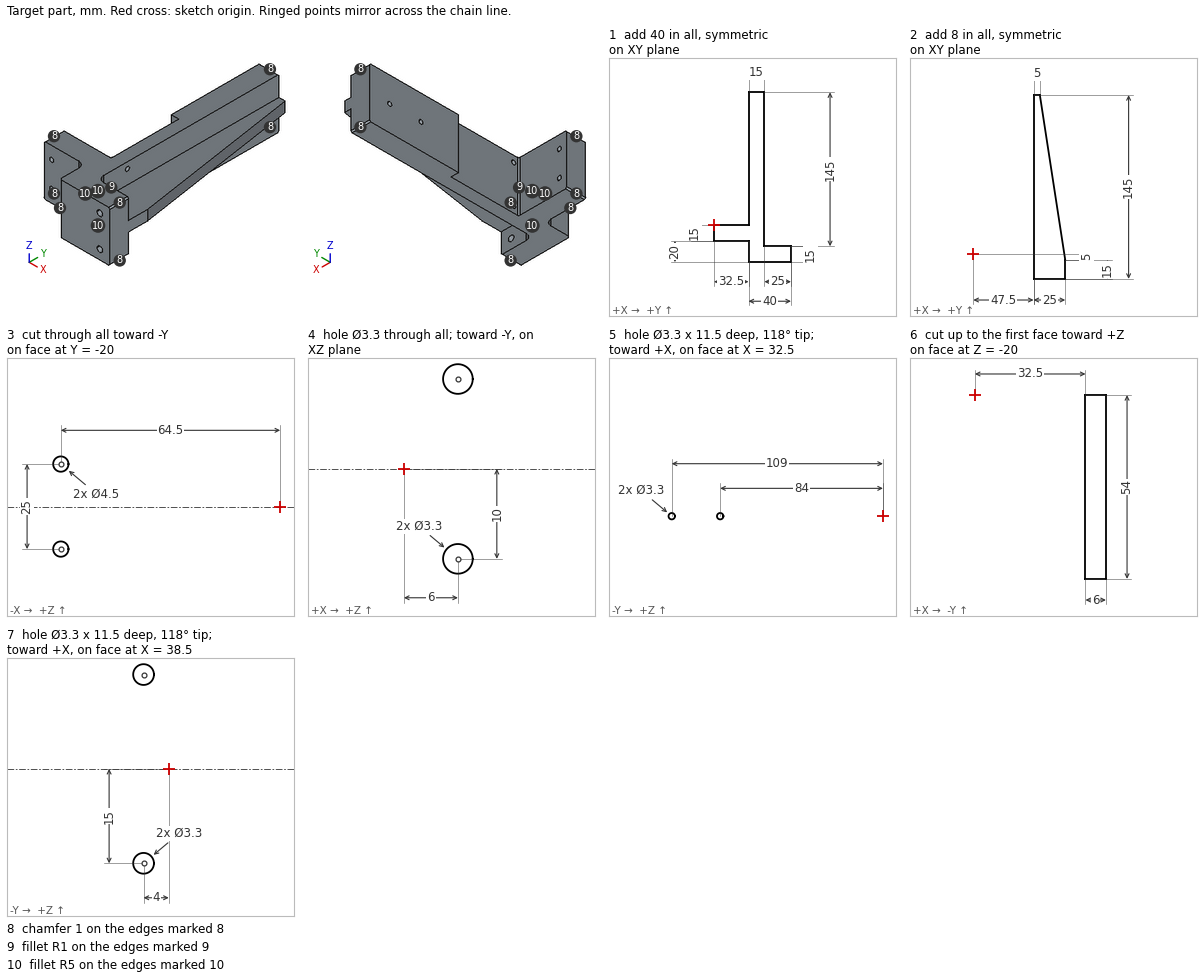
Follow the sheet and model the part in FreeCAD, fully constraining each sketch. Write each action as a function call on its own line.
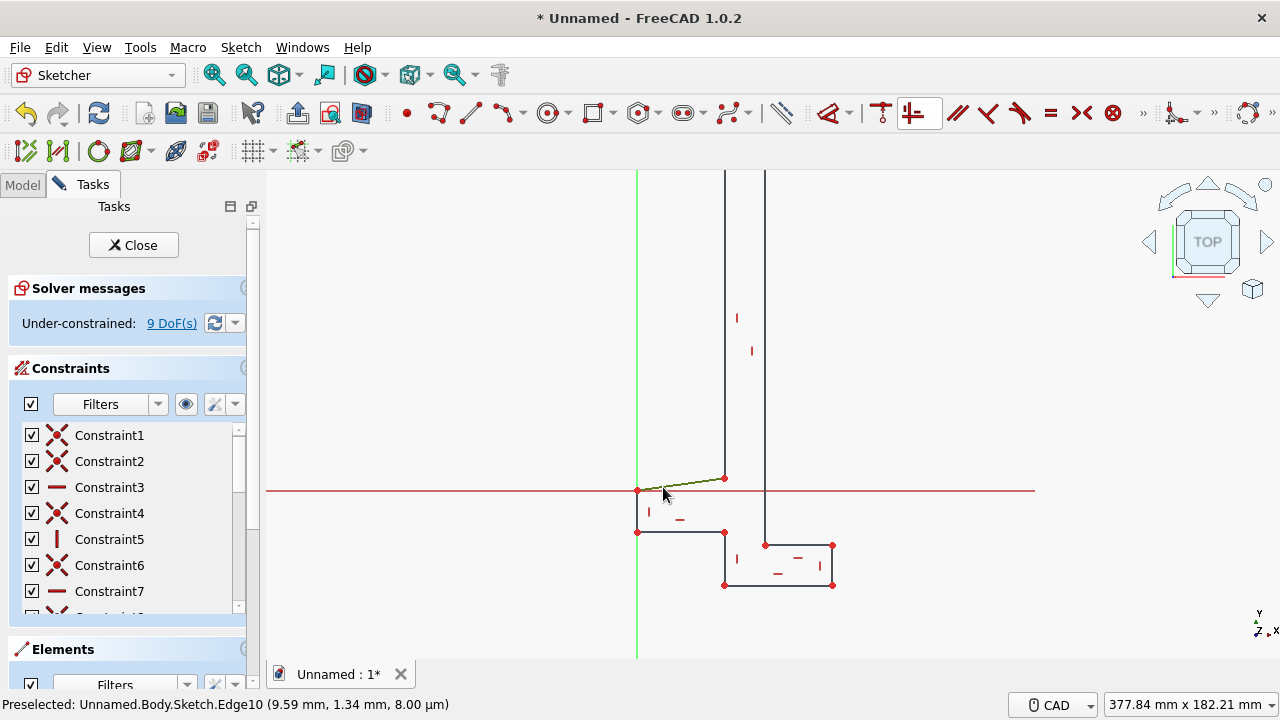
key(h)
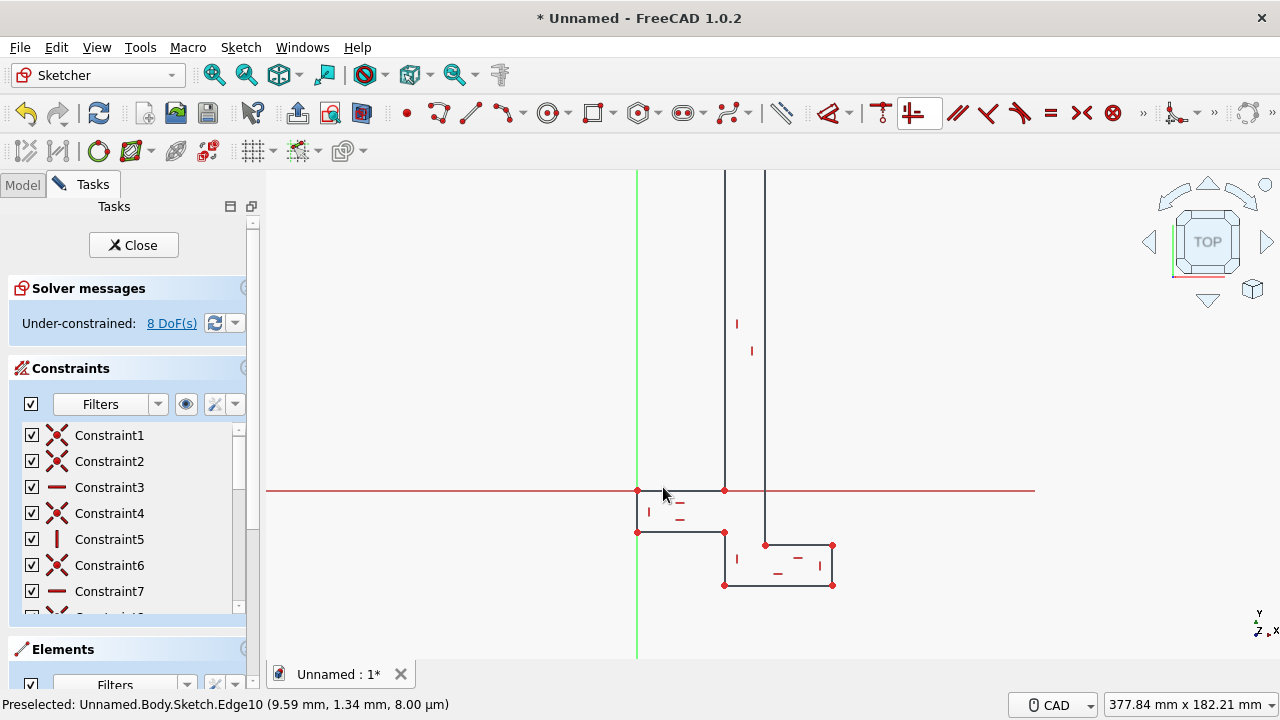
key(d)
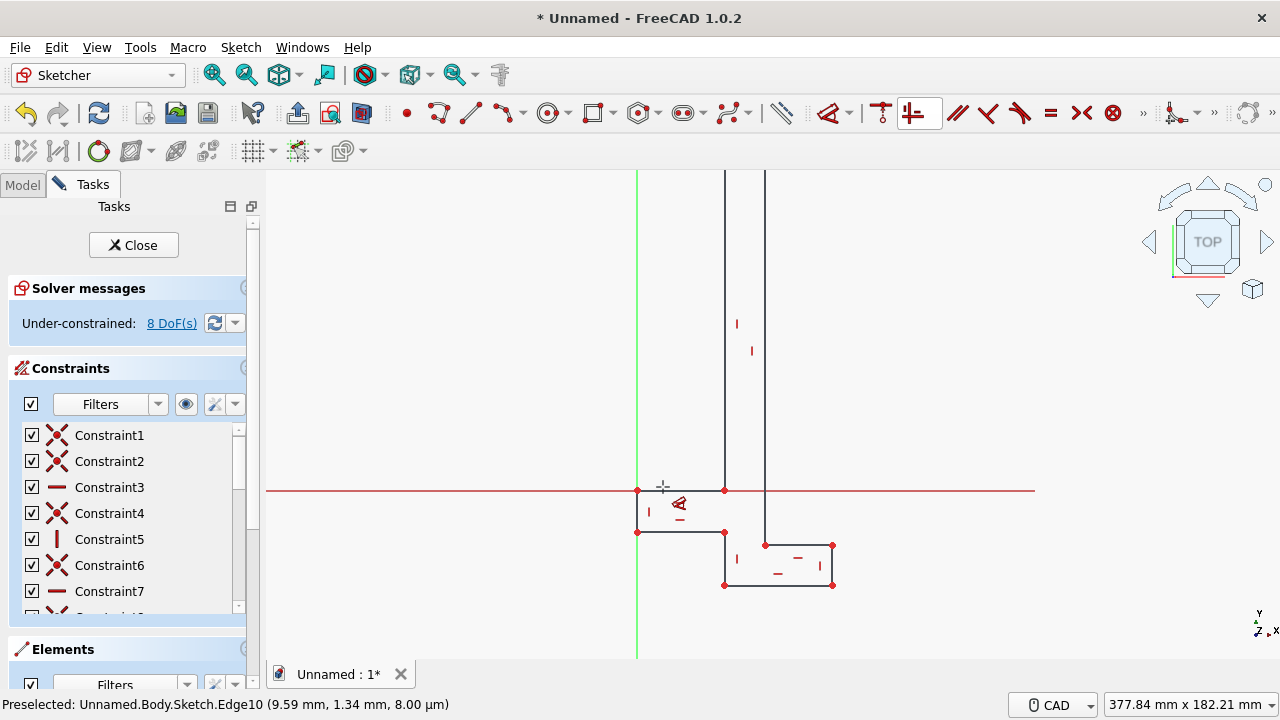
click(637, 503)
click(603, 511)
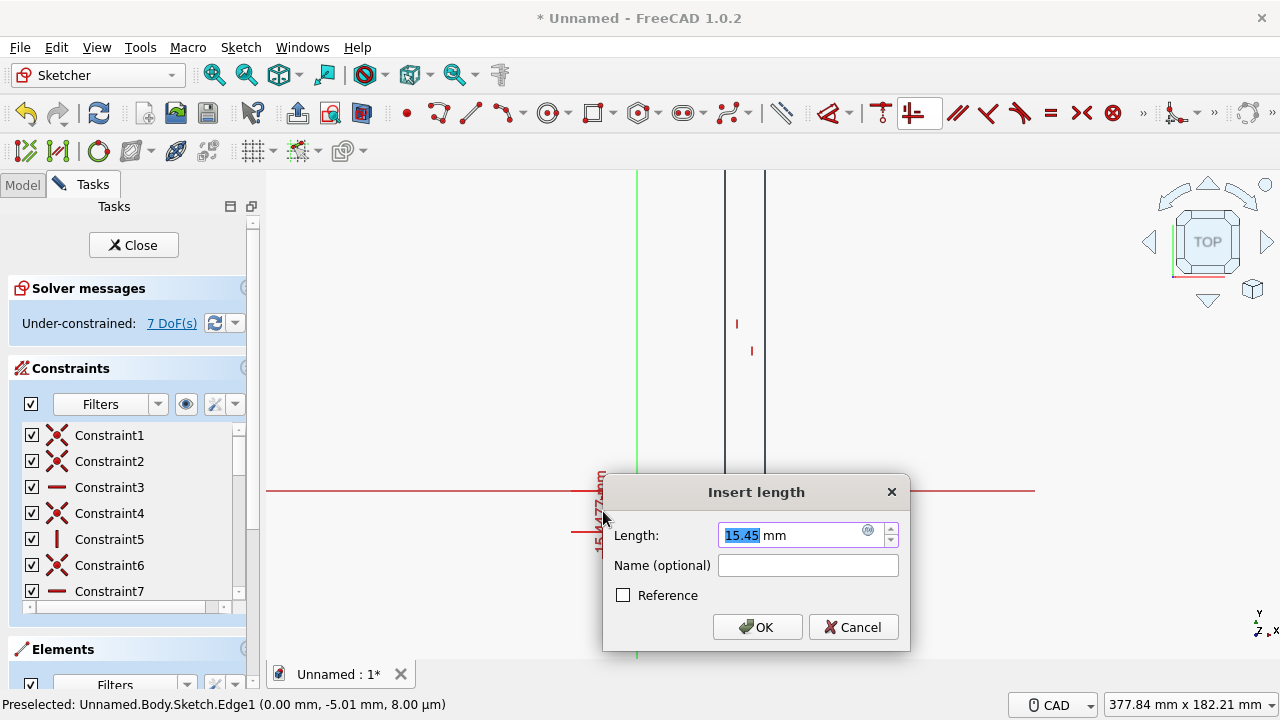
text(15)
key(Return)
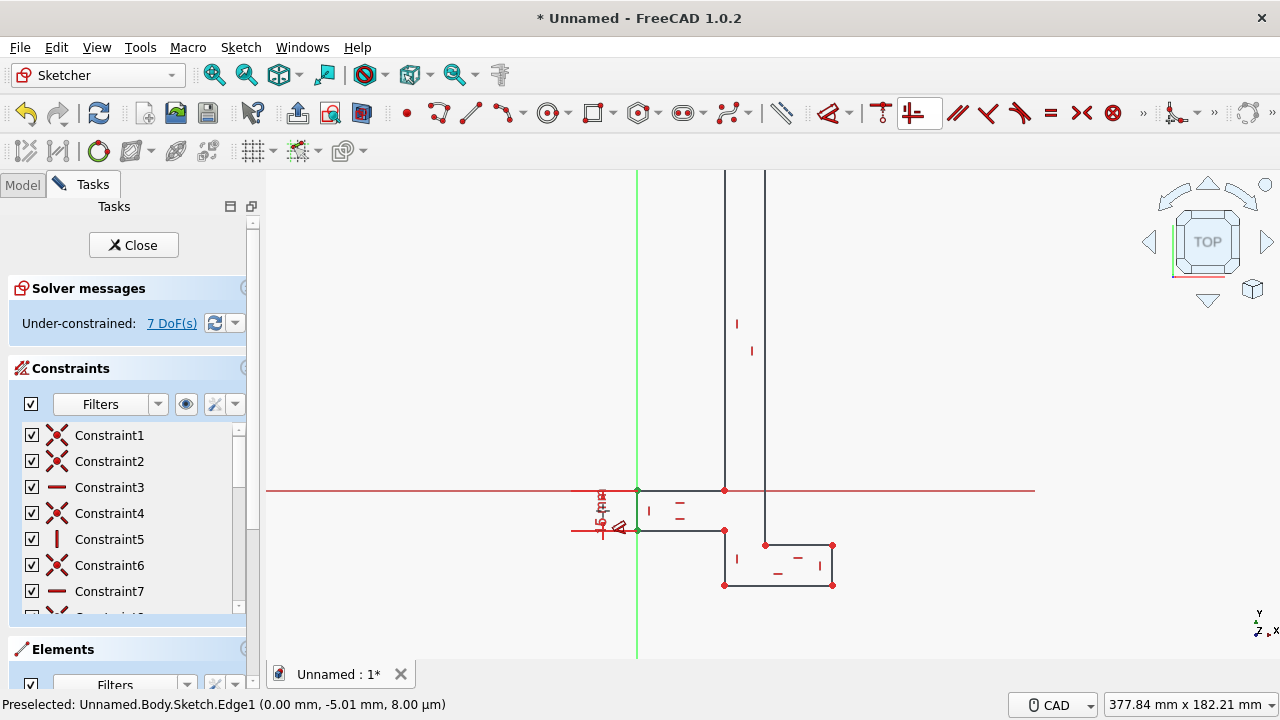
click(725, 547)
click(691, 558)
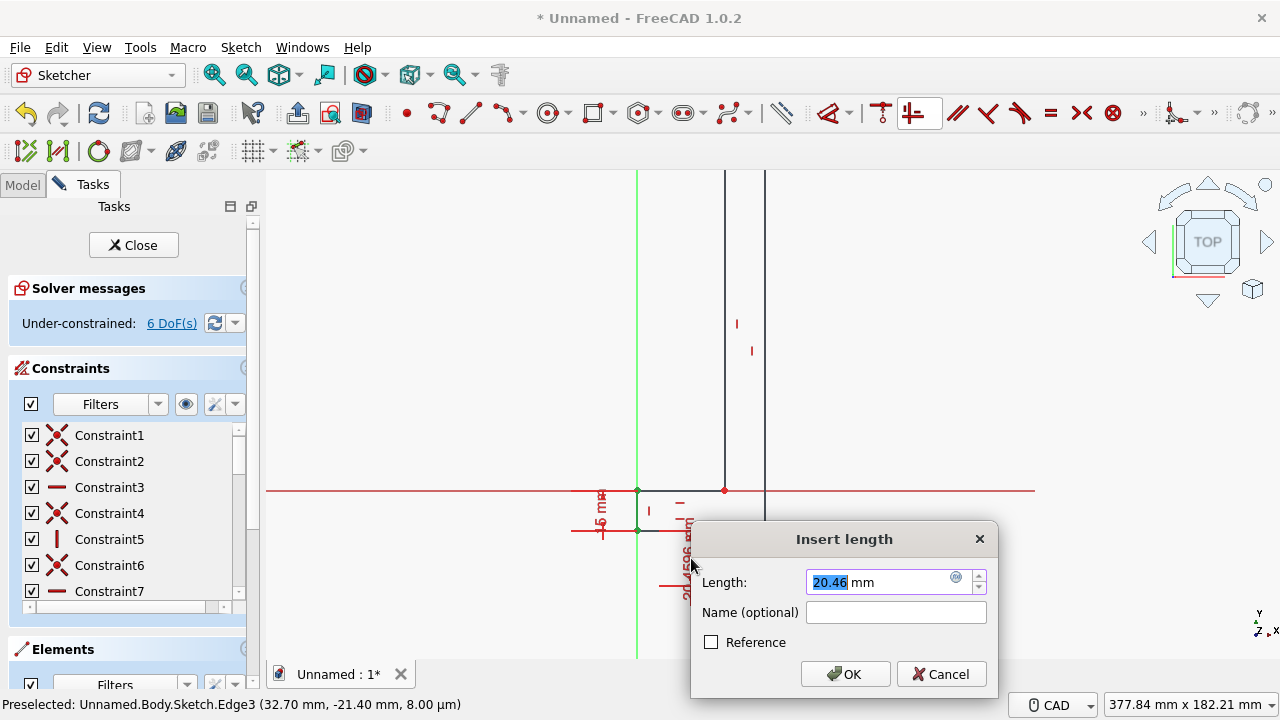
text(20)
key(Return)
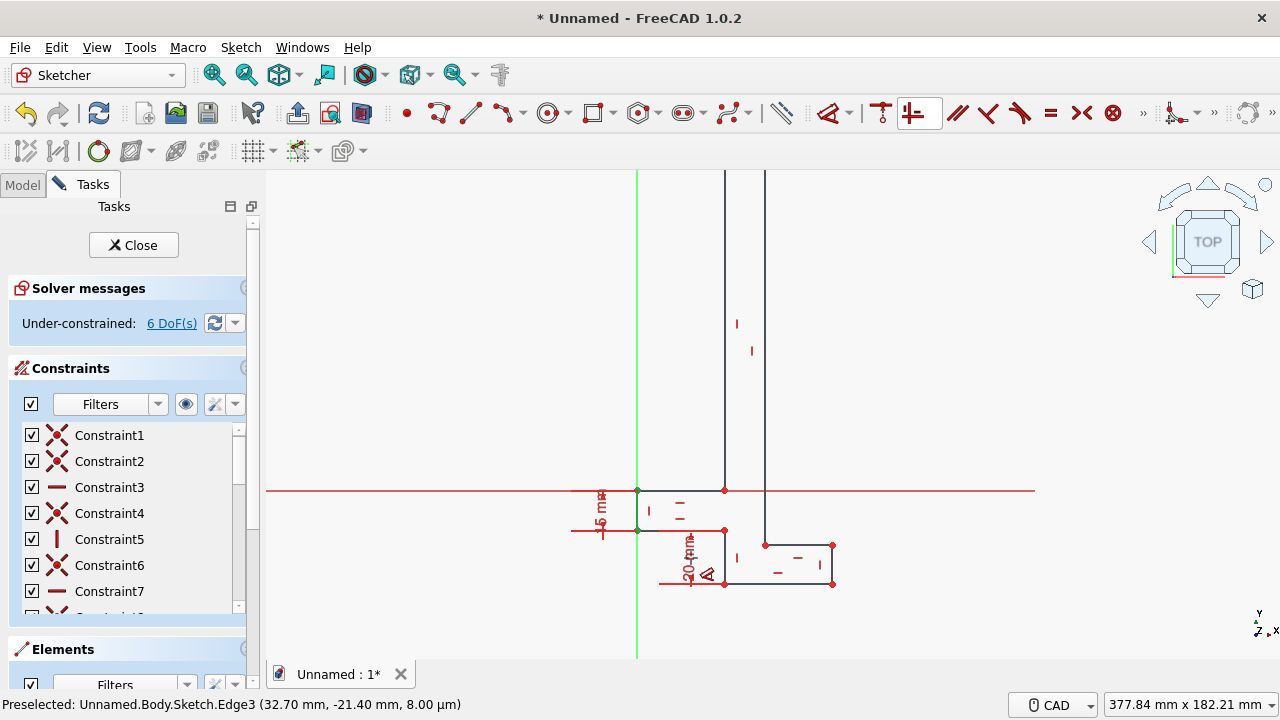
click(757, 584)
click(779, 618)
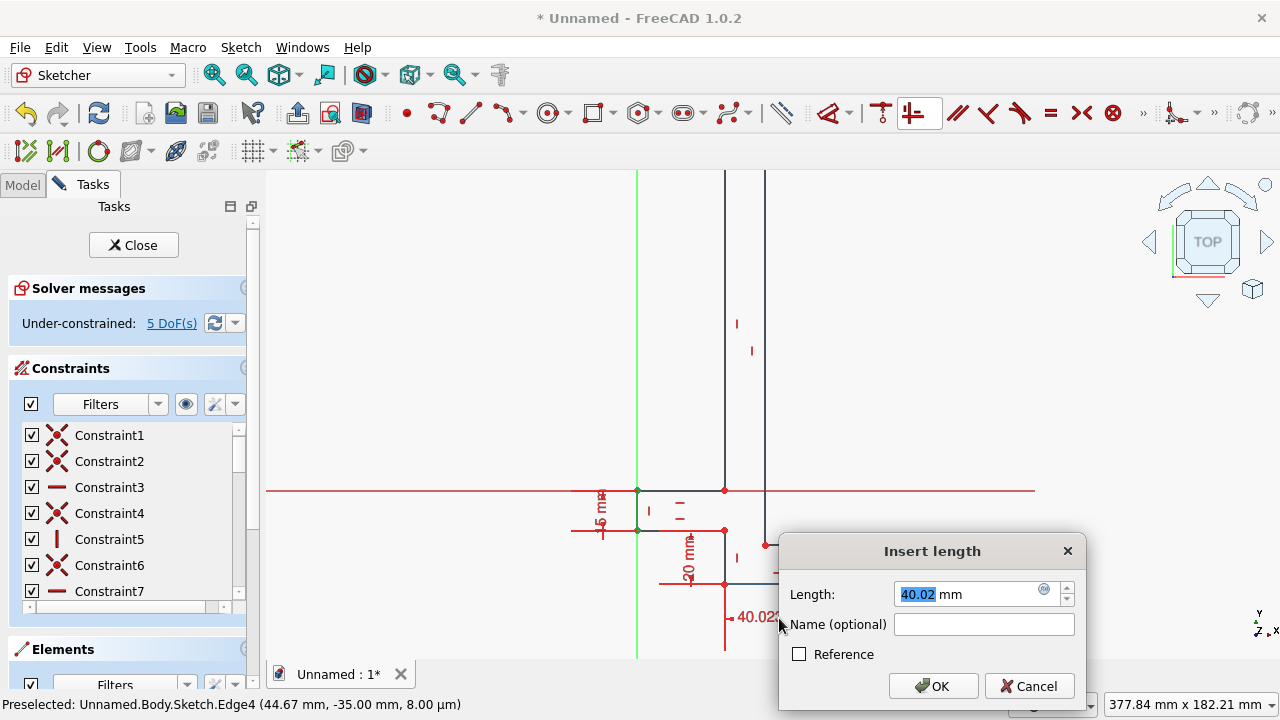
text(40)
key(Return)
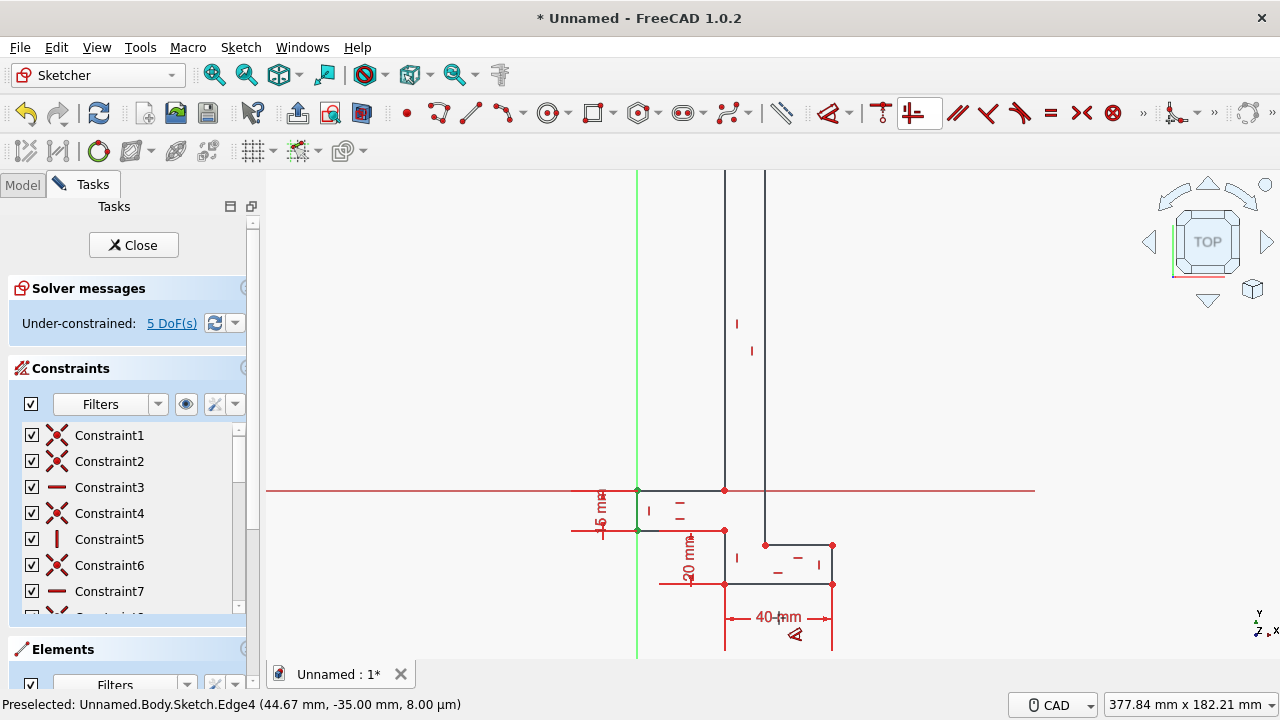
click(832, 573)
click(866, 565)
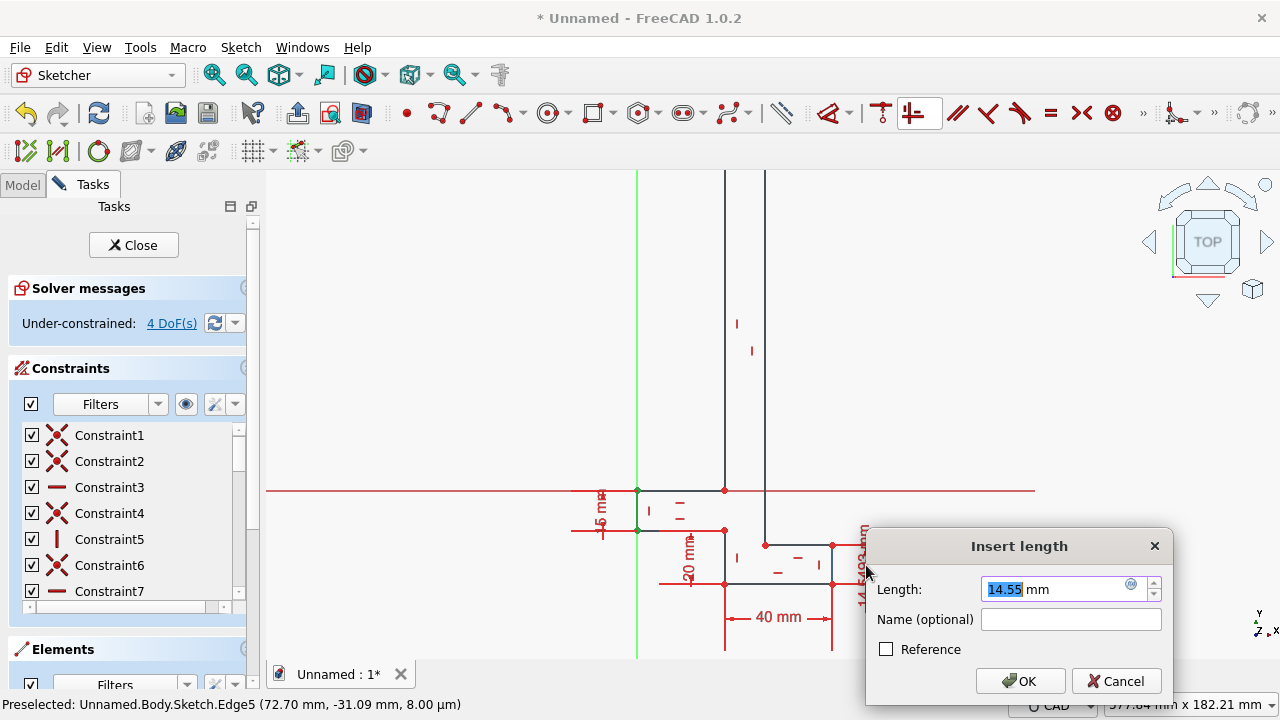
text(15)
key(Return)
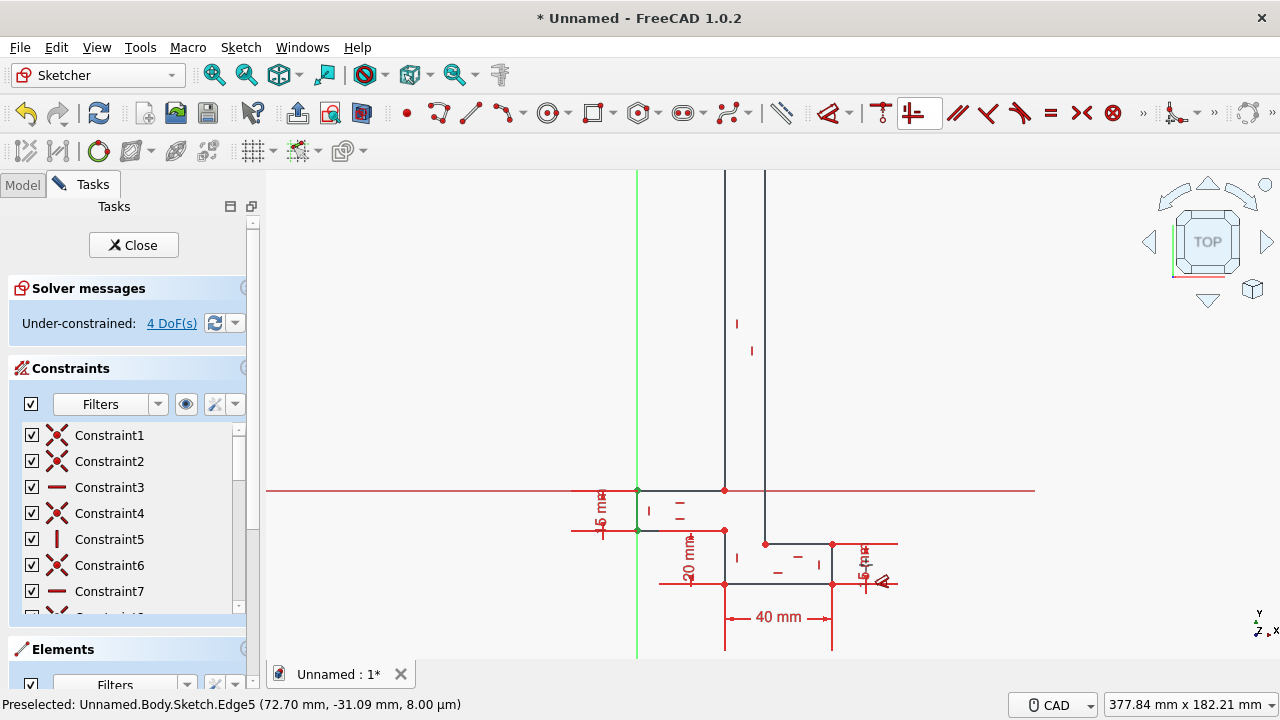
click(812, 544)
click(799, 510)